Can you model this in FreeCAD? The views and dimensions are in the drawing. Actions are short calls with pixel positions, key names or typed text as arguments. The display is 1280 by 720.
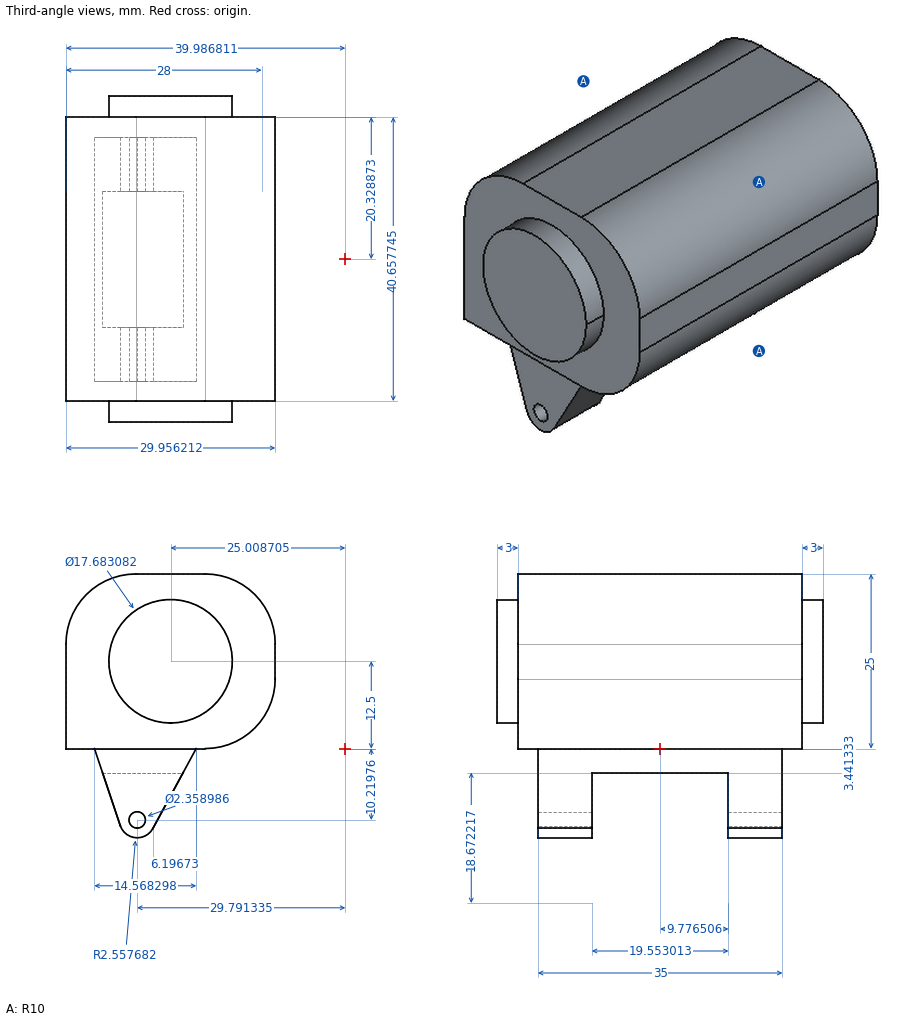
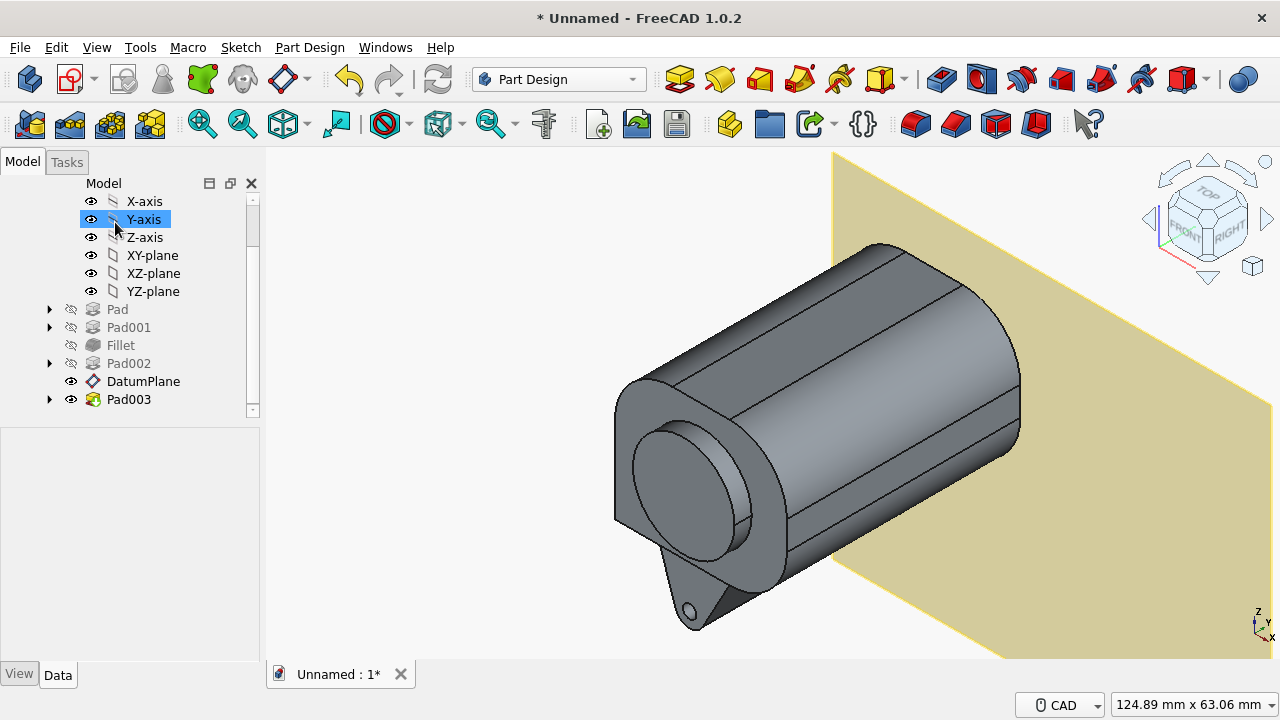
click(116, 381)
key(space)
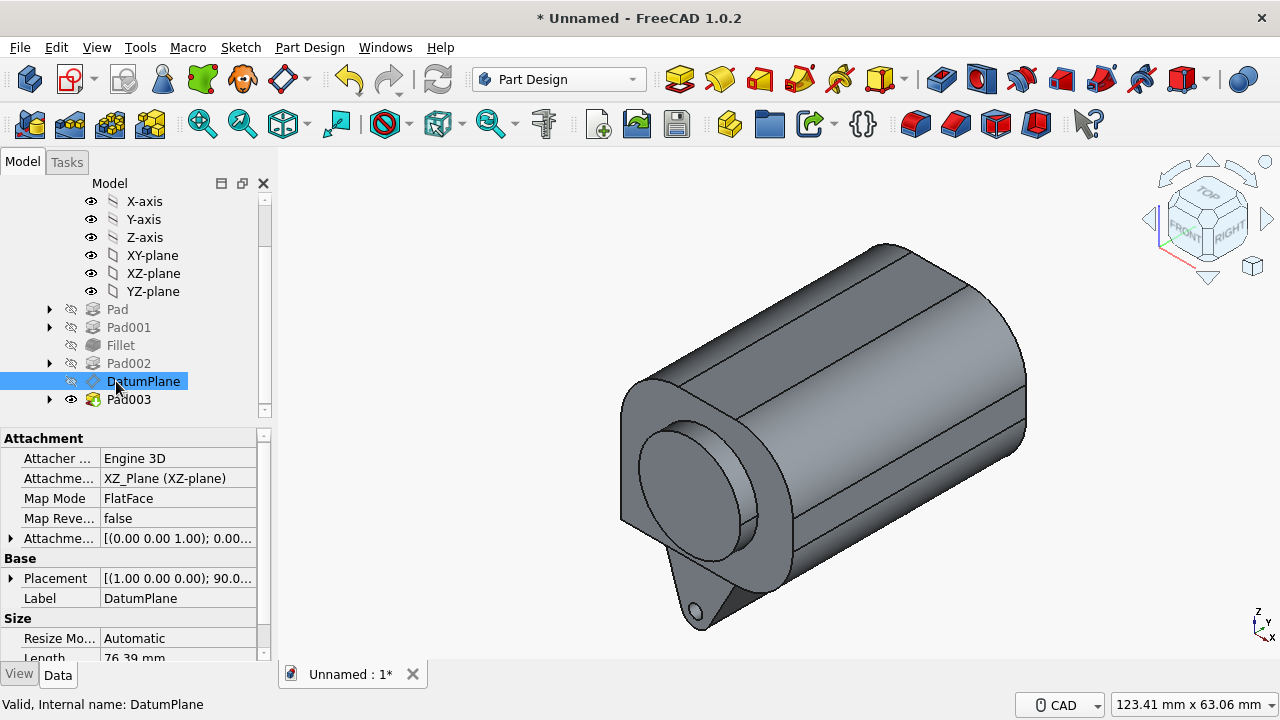
click(204, 124)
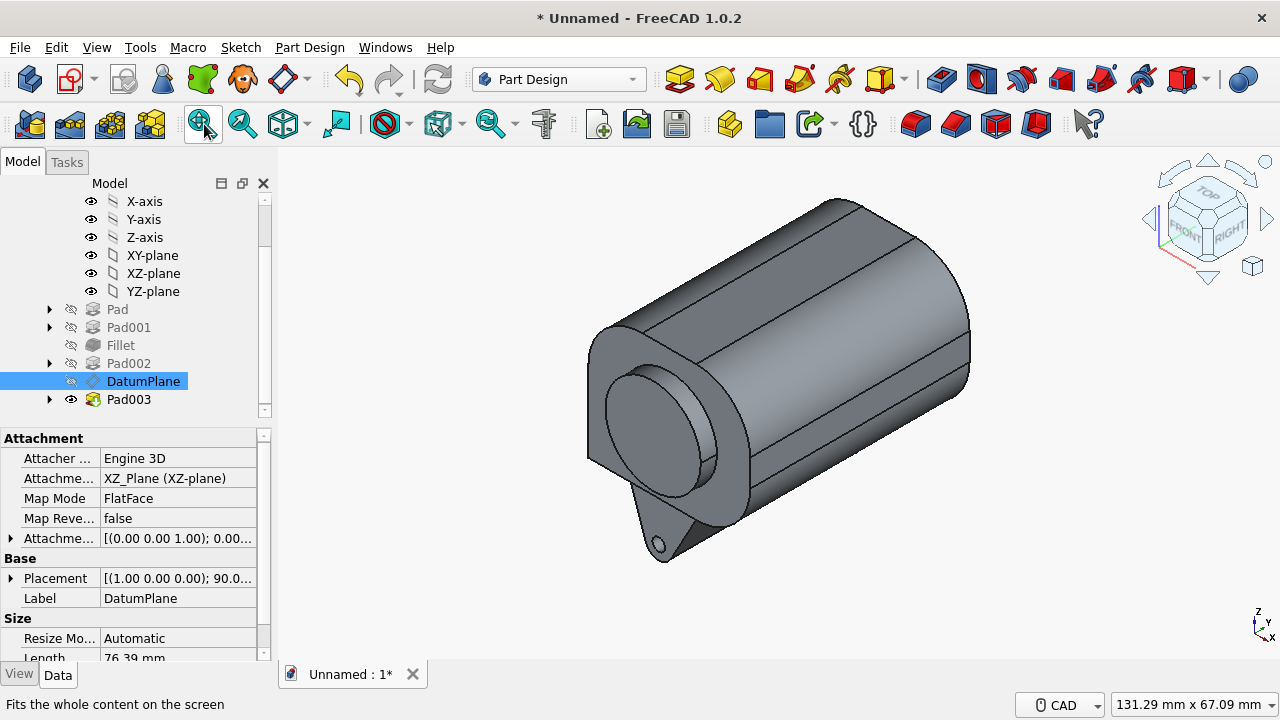
key(6)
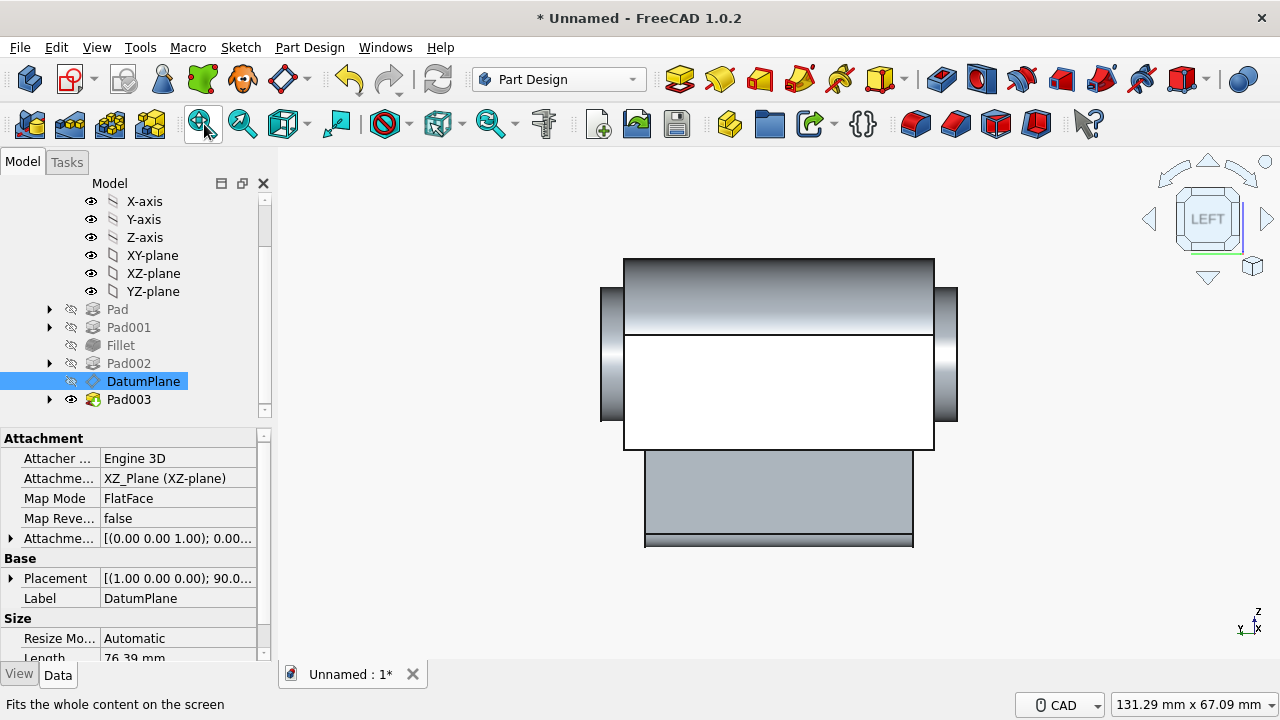
click(690, 391)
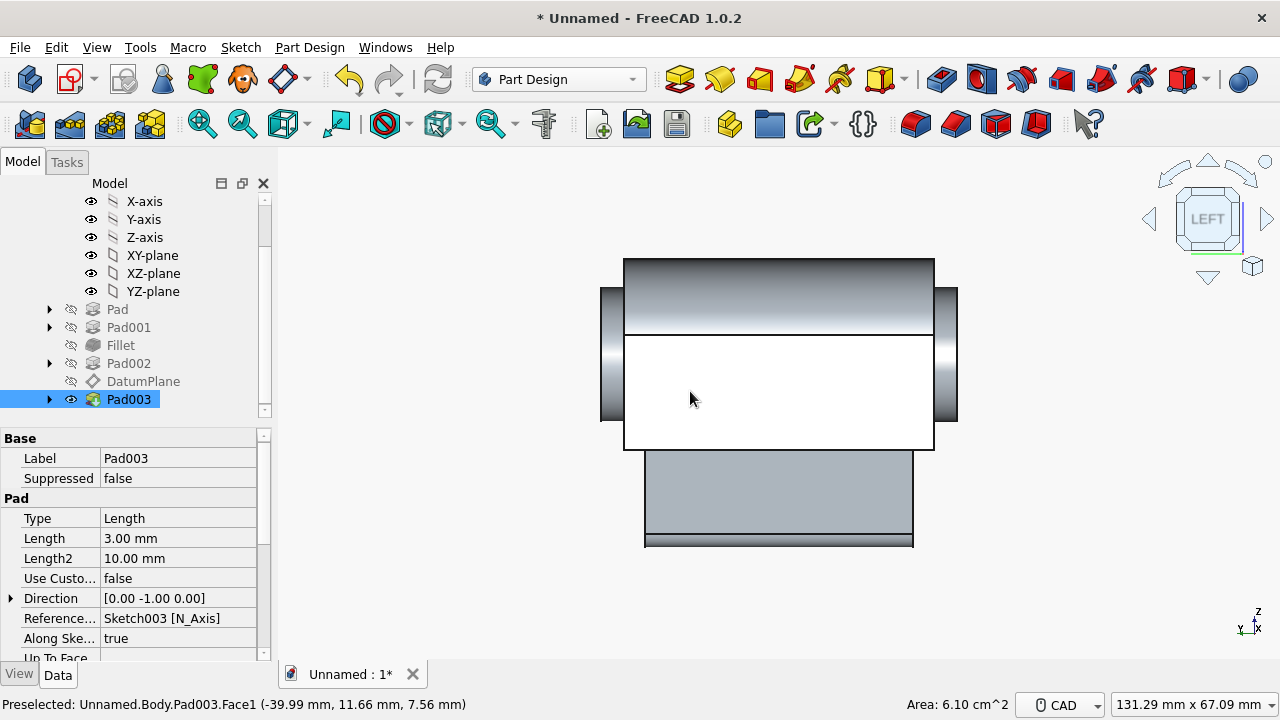
click(70, 80)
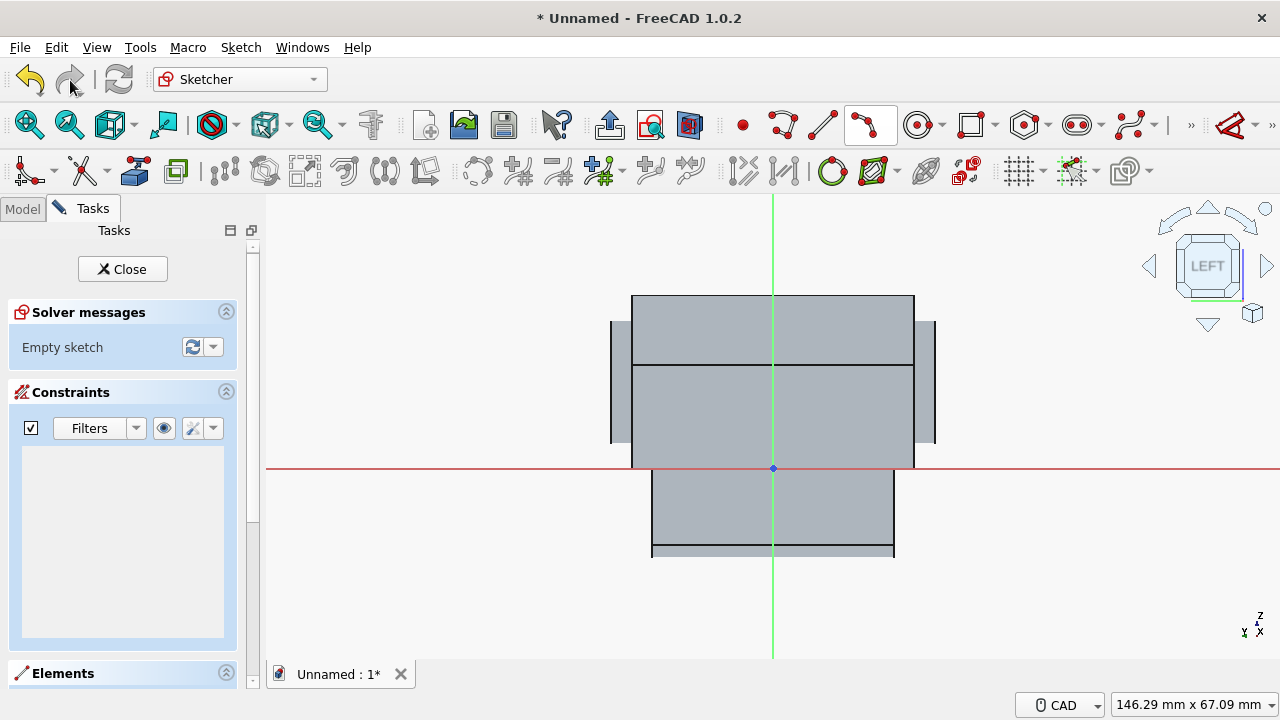
scroll(704, 426, down, 5)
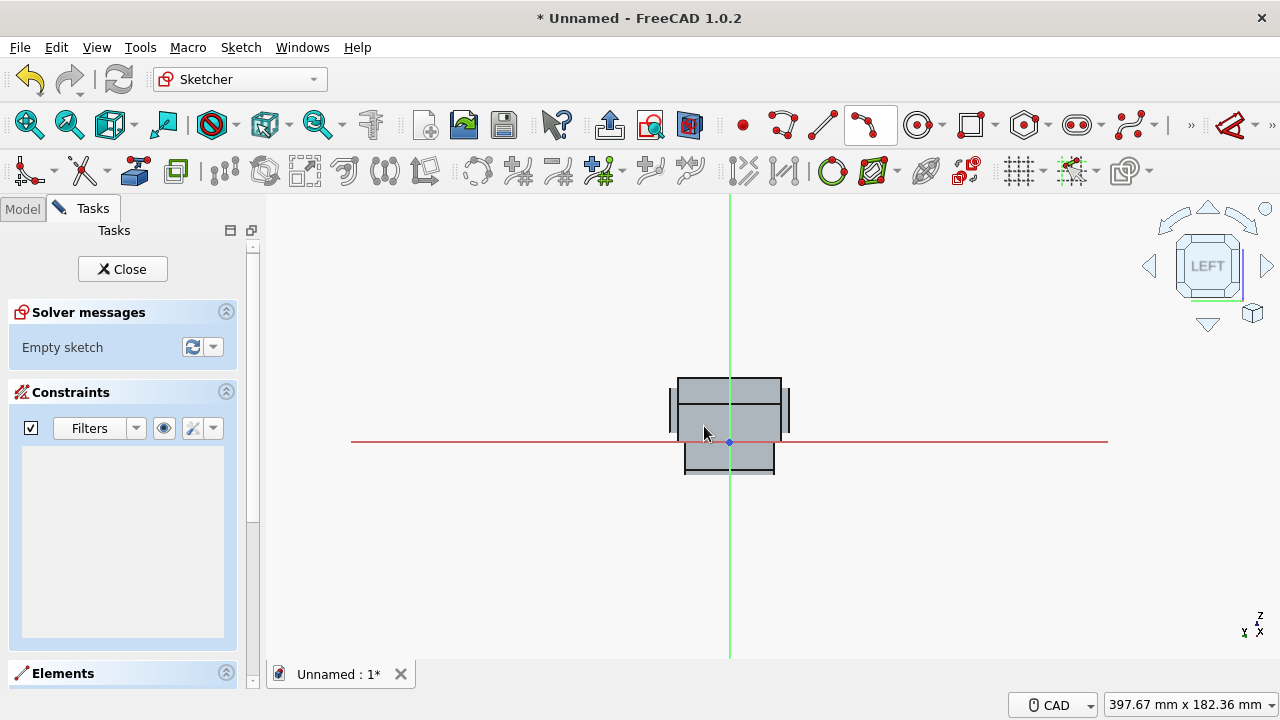
scroll(736, 481, up, 8)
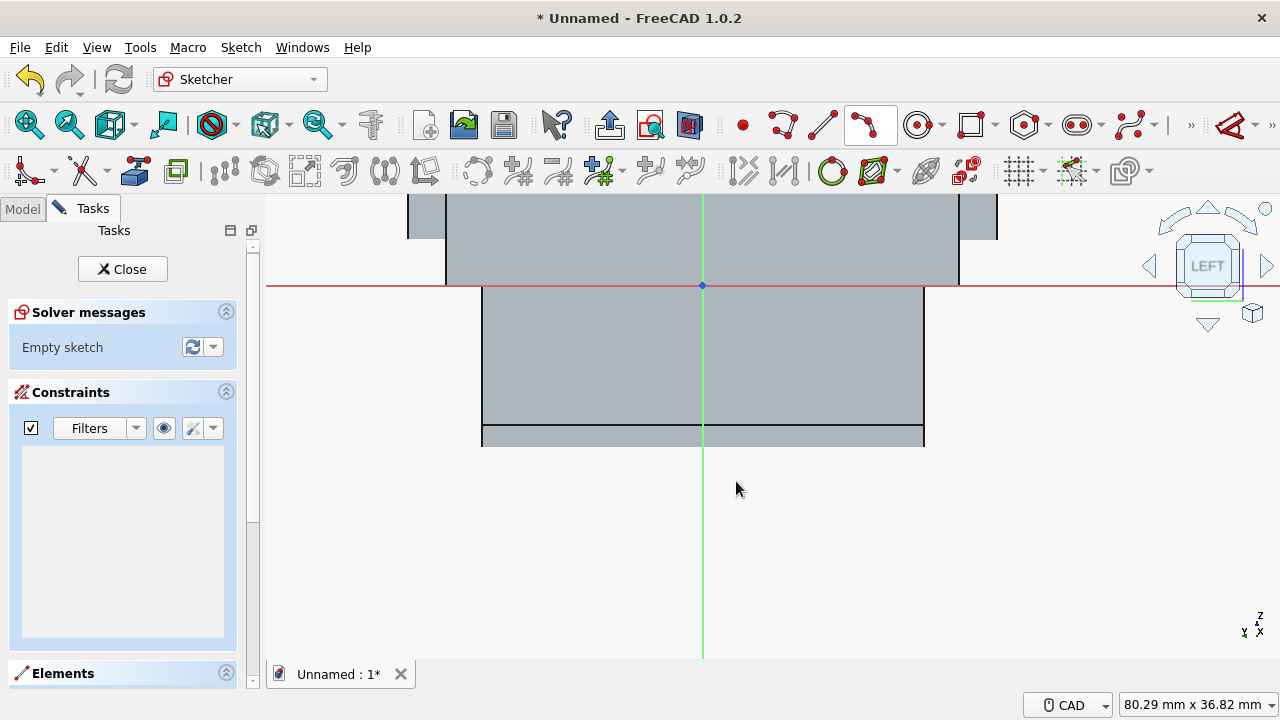
click(972, 126)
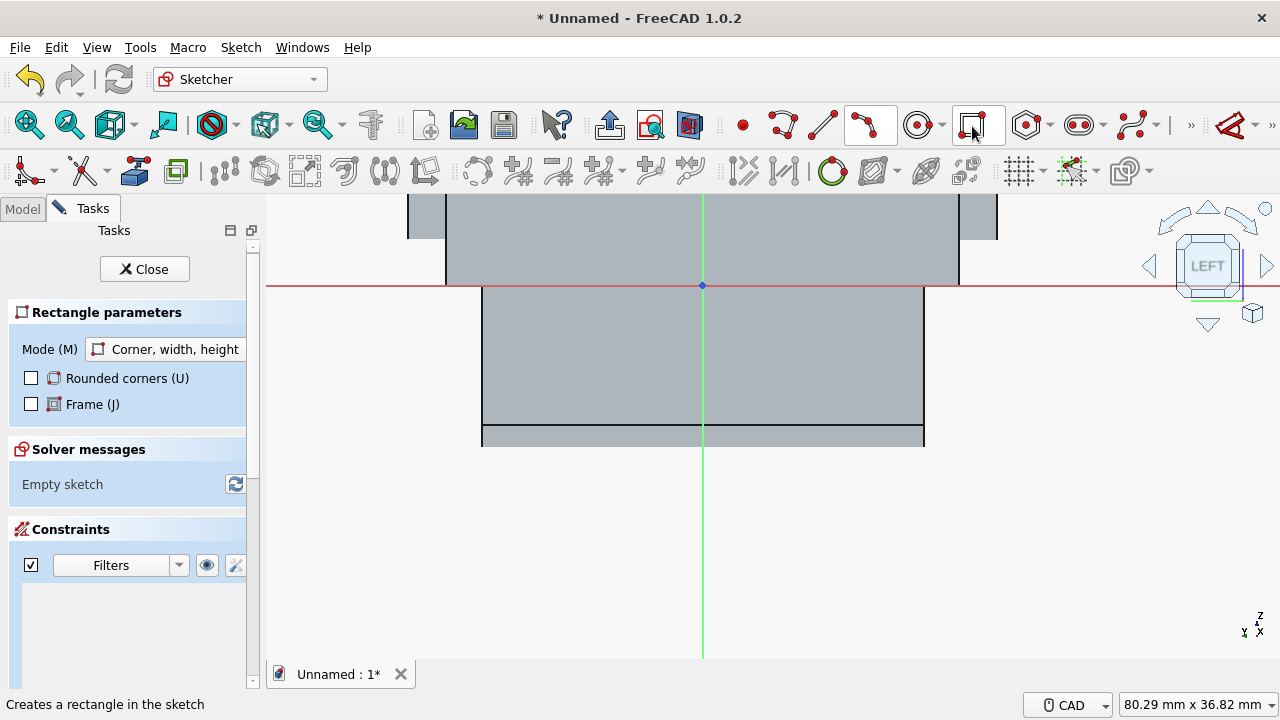
click(579, 329)
move(826, 565)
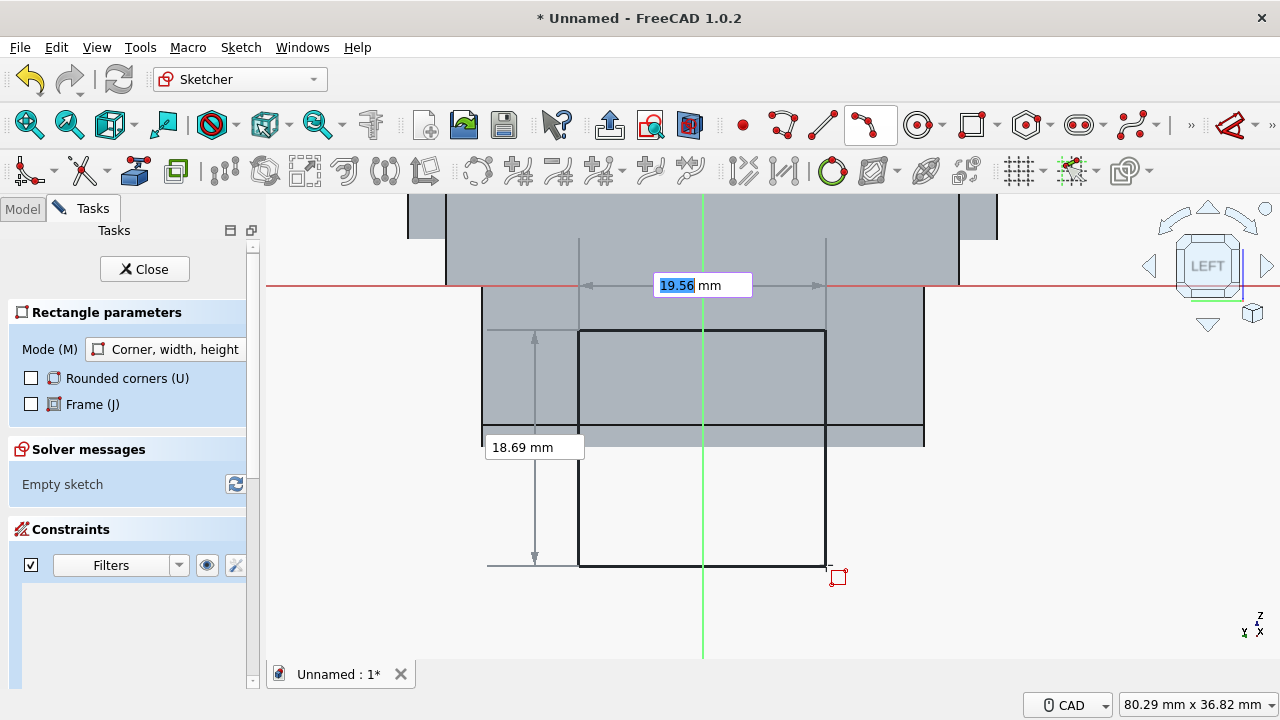
text(19.553013)
key(Tab)
text(18.672217)
key(Return)
key(Escape)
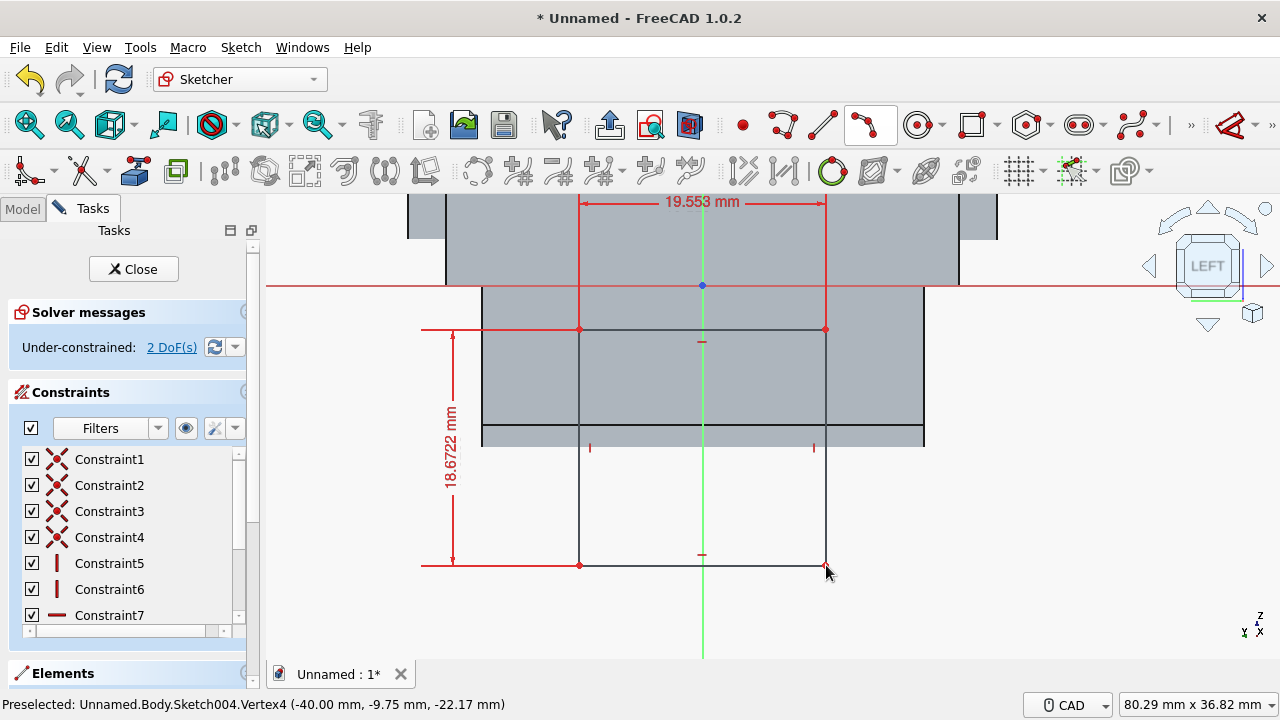
click(1230, 126)